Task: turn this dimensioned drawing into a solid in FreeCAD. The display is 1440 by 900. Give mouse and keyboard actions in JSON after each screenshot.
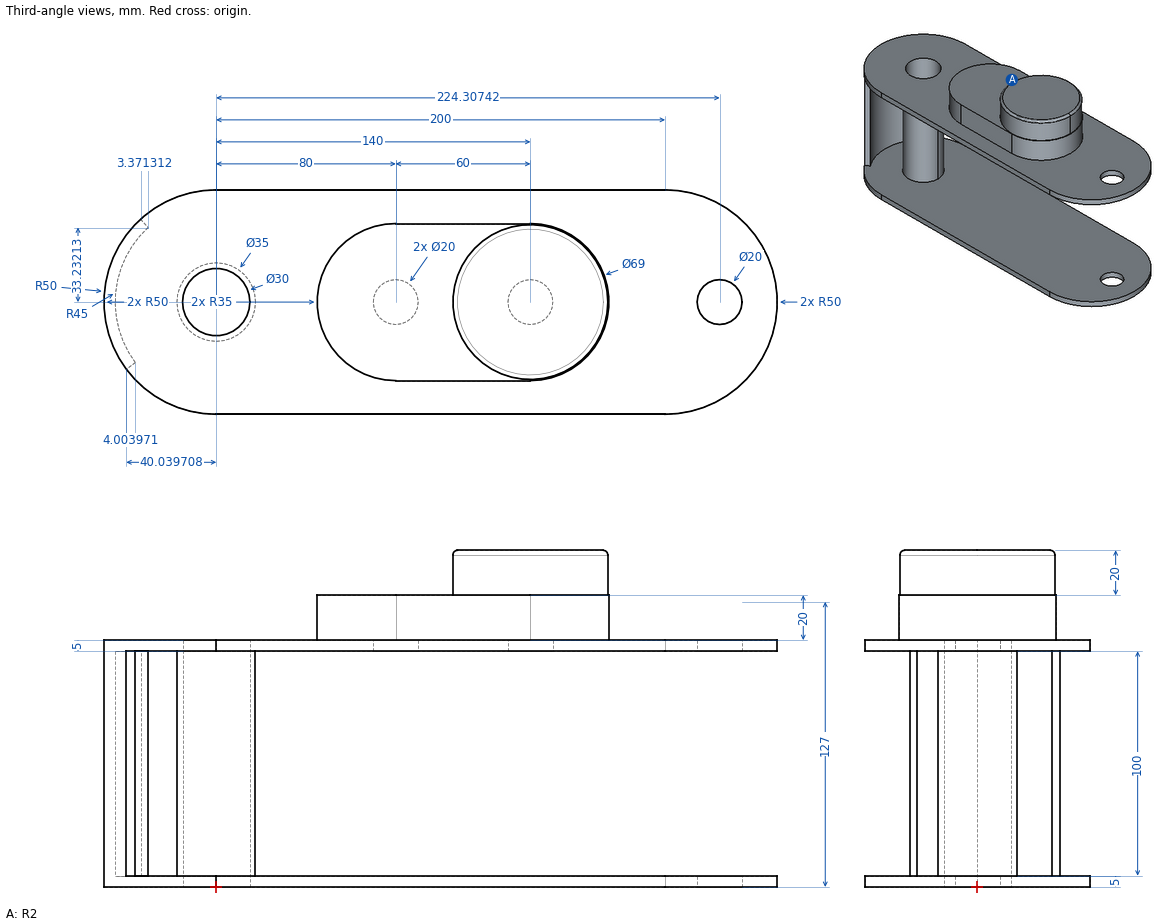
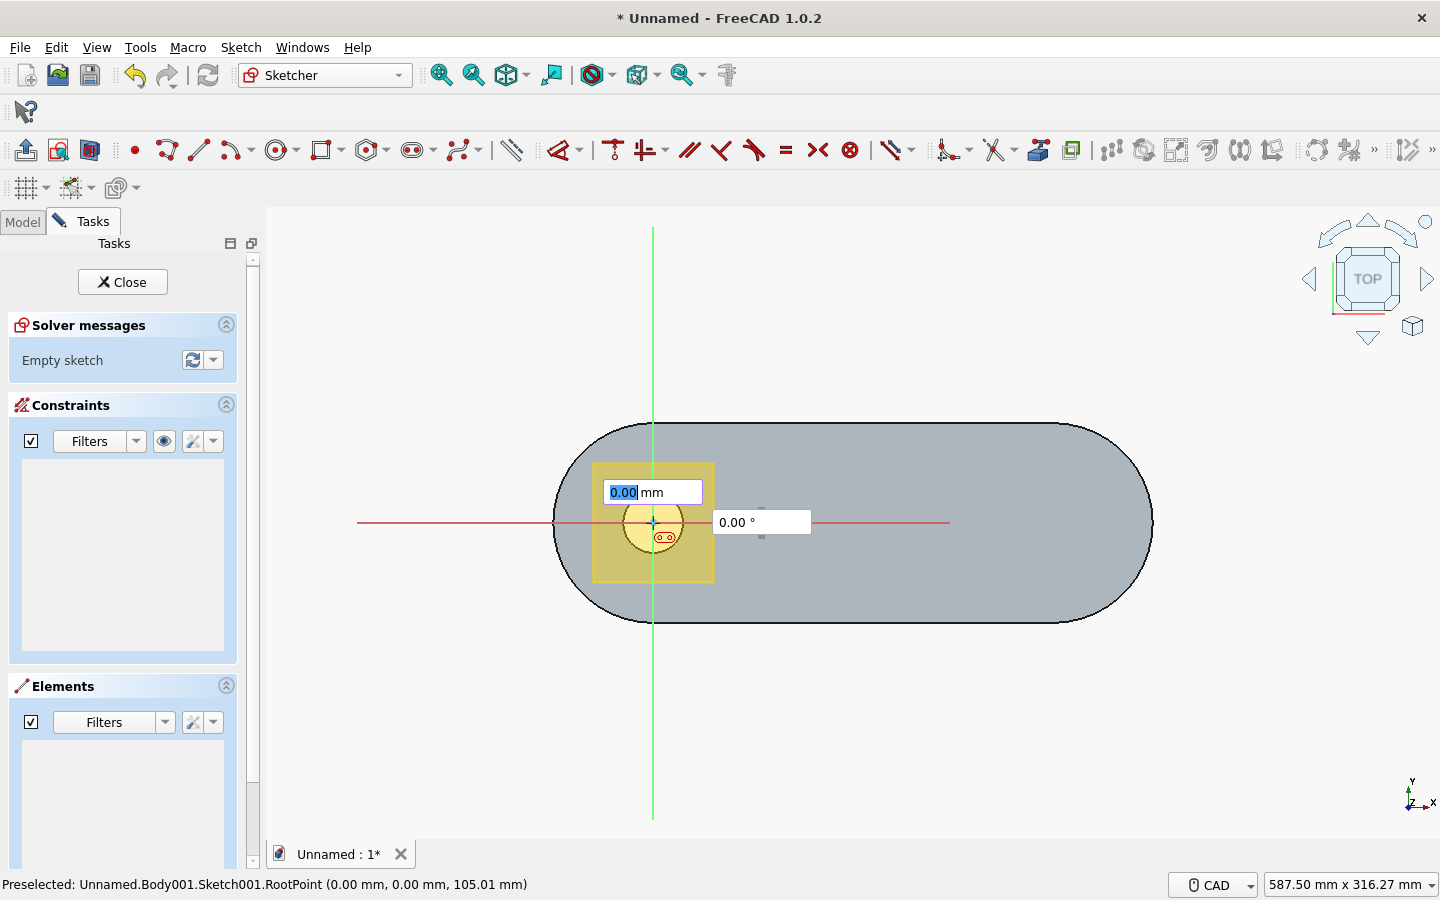
{"action": "left_click", "coordinate": [1053, 514]}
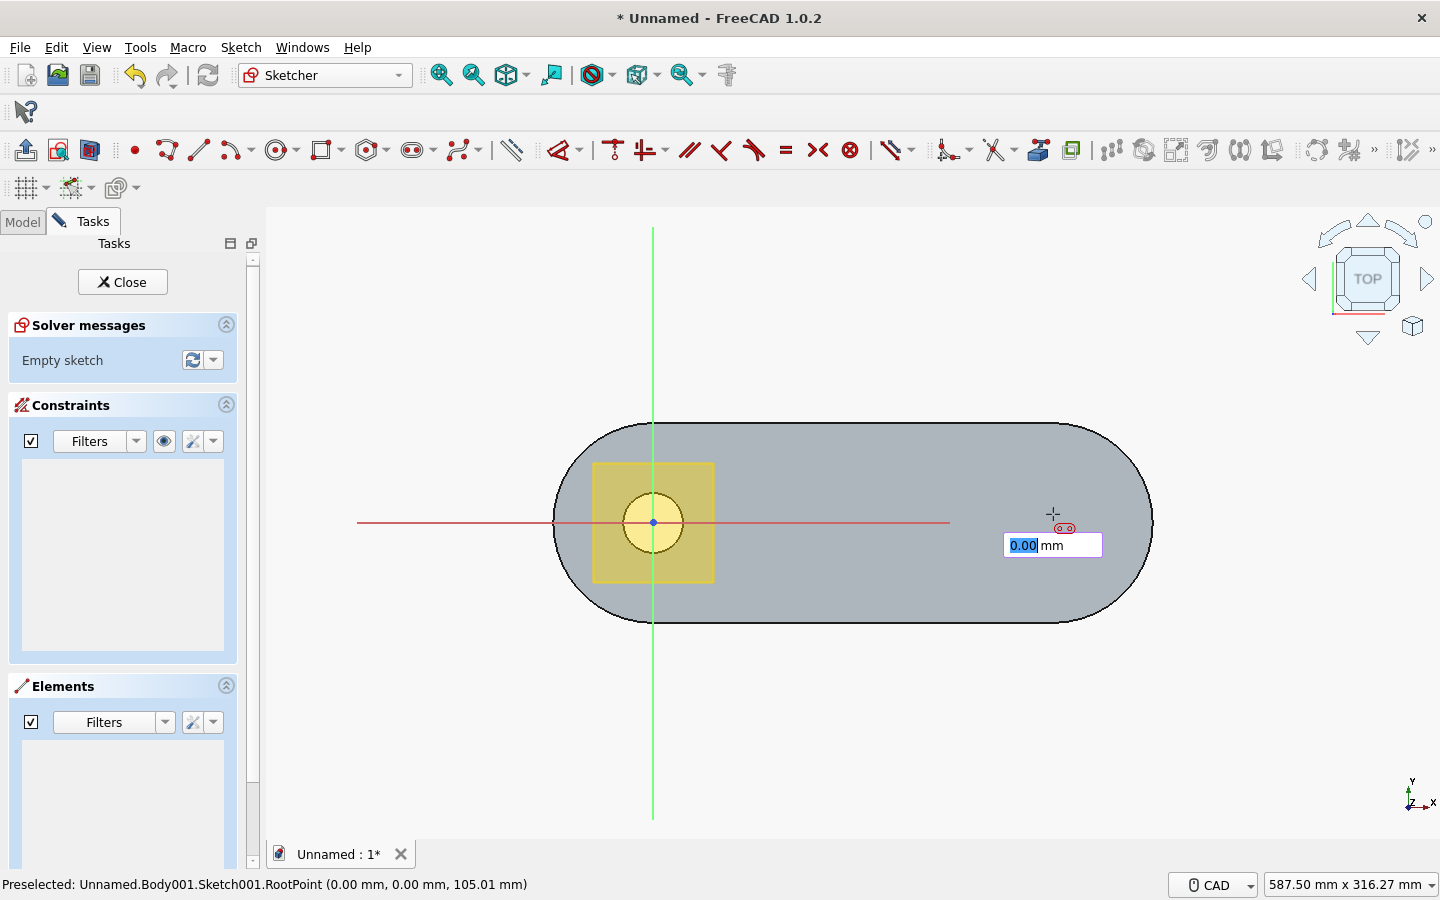
{"action": "left_click", "coordinate": [853, 623]}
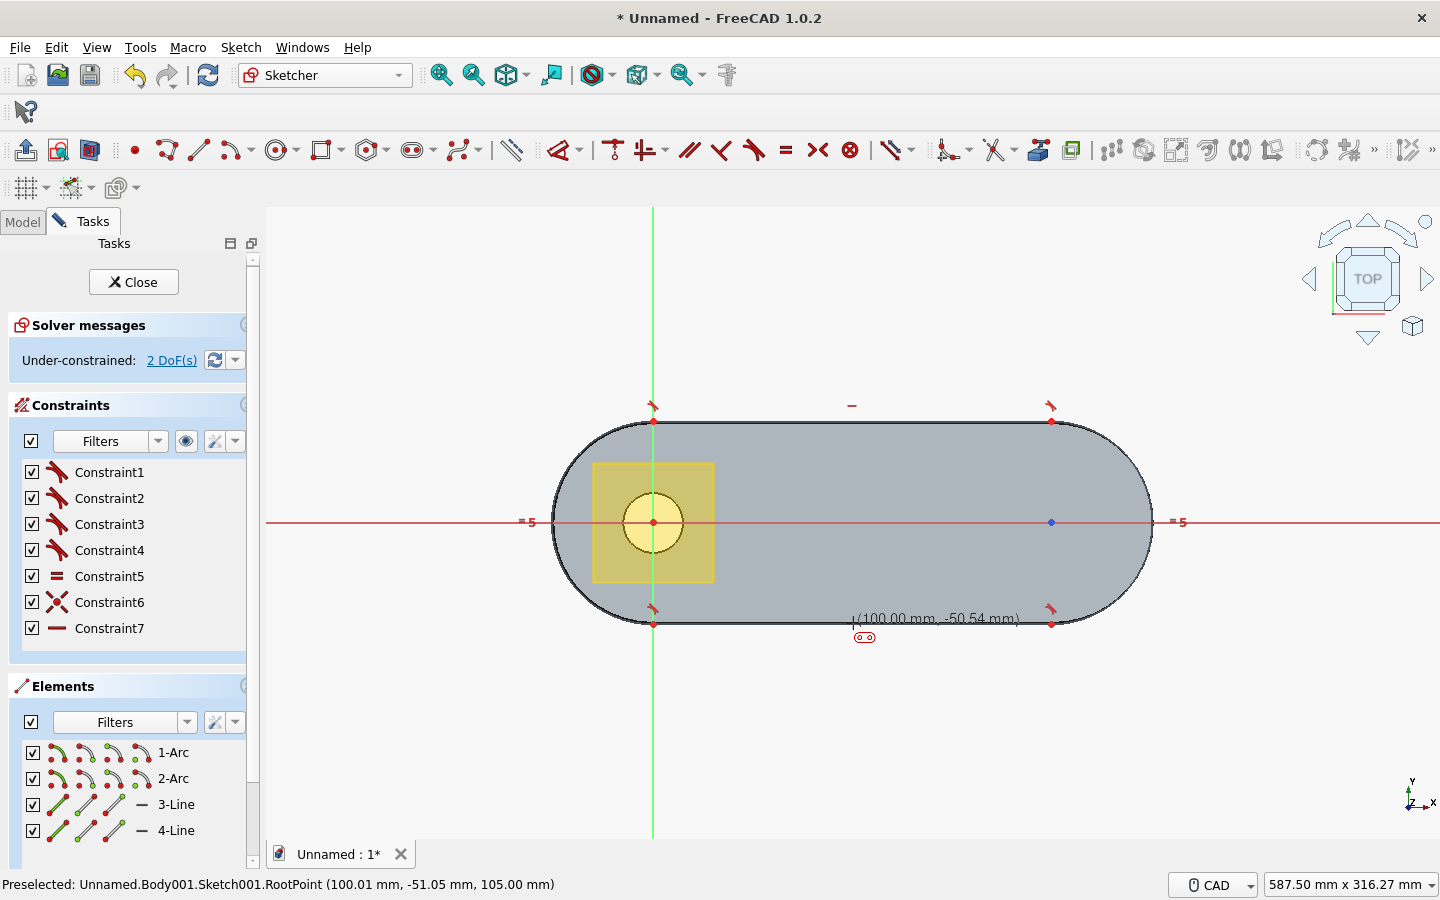
{"action": "left_click", "coordinate": [276, 150]}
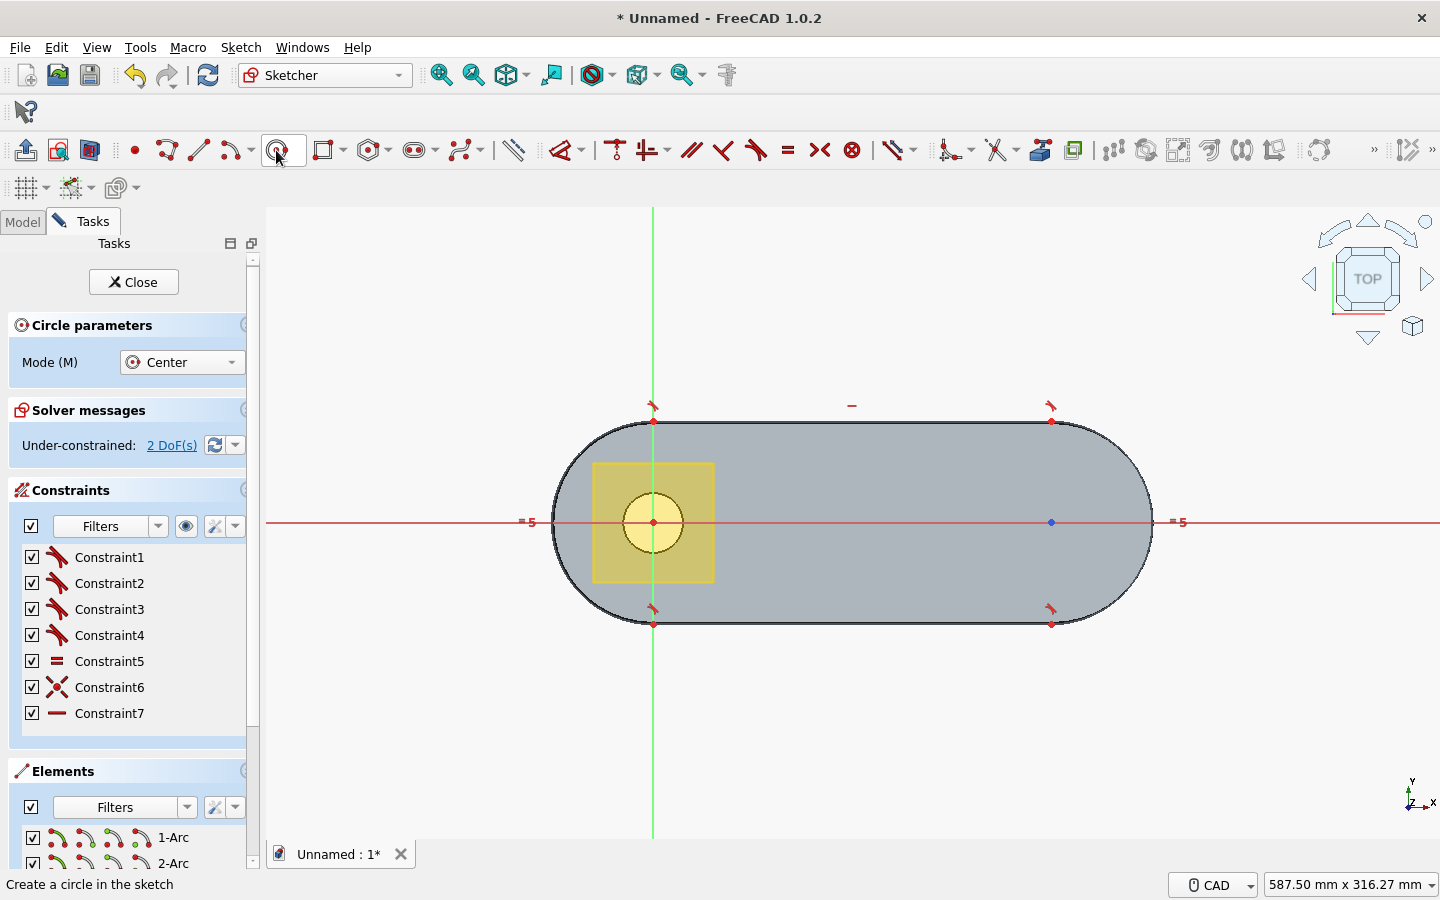
{"action": "left_click", "coordinate": [653, 523]}
{"action": "left_click", "coordinate": [674, 502]}
{"action": "key", "text": "Escape"}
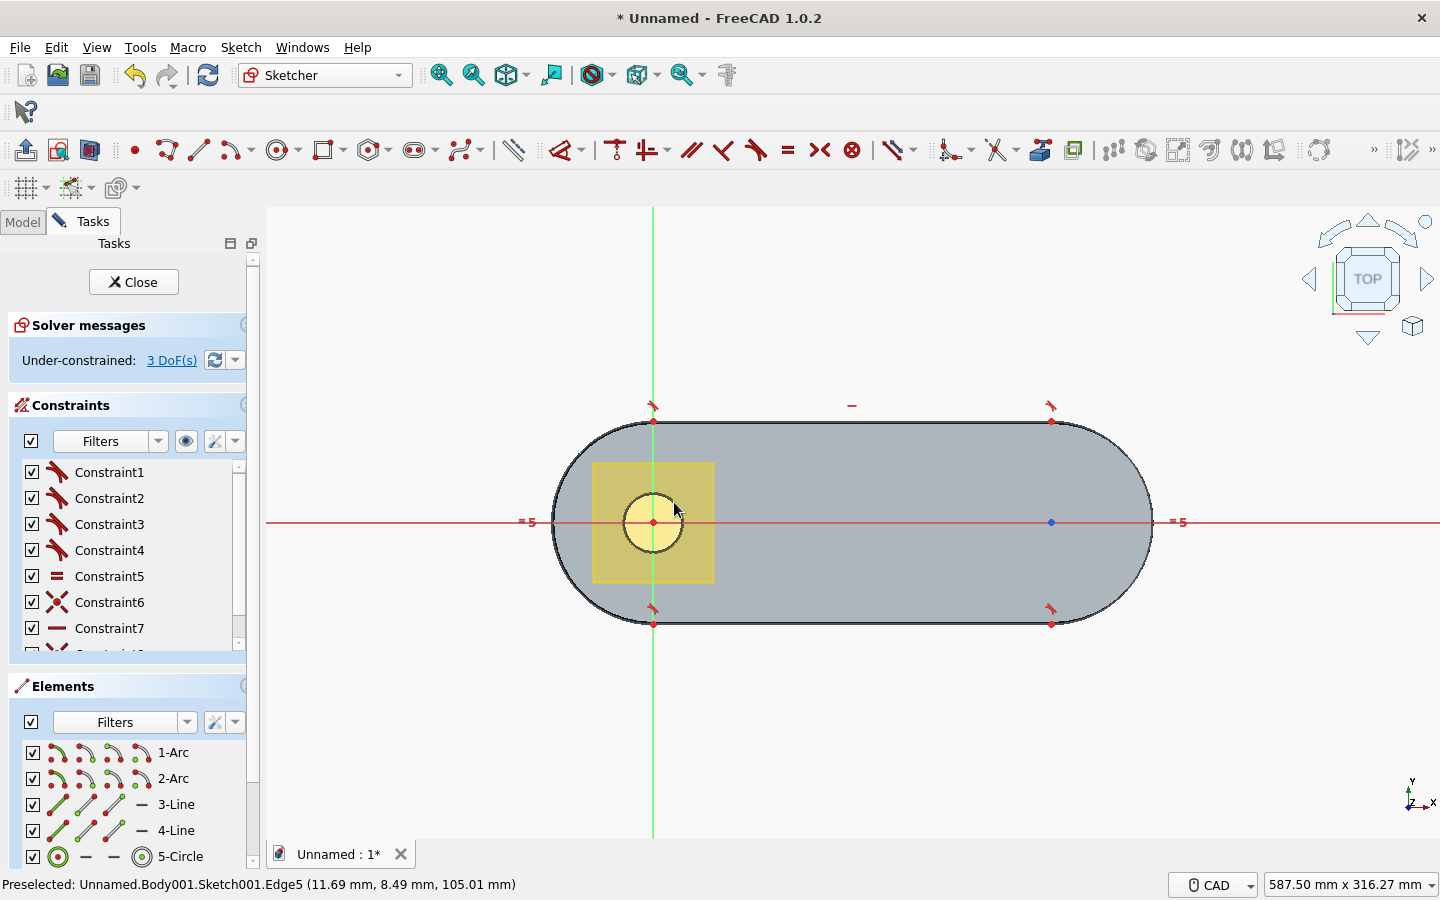
{"action": "left_click", "coordinate": [560, 150]}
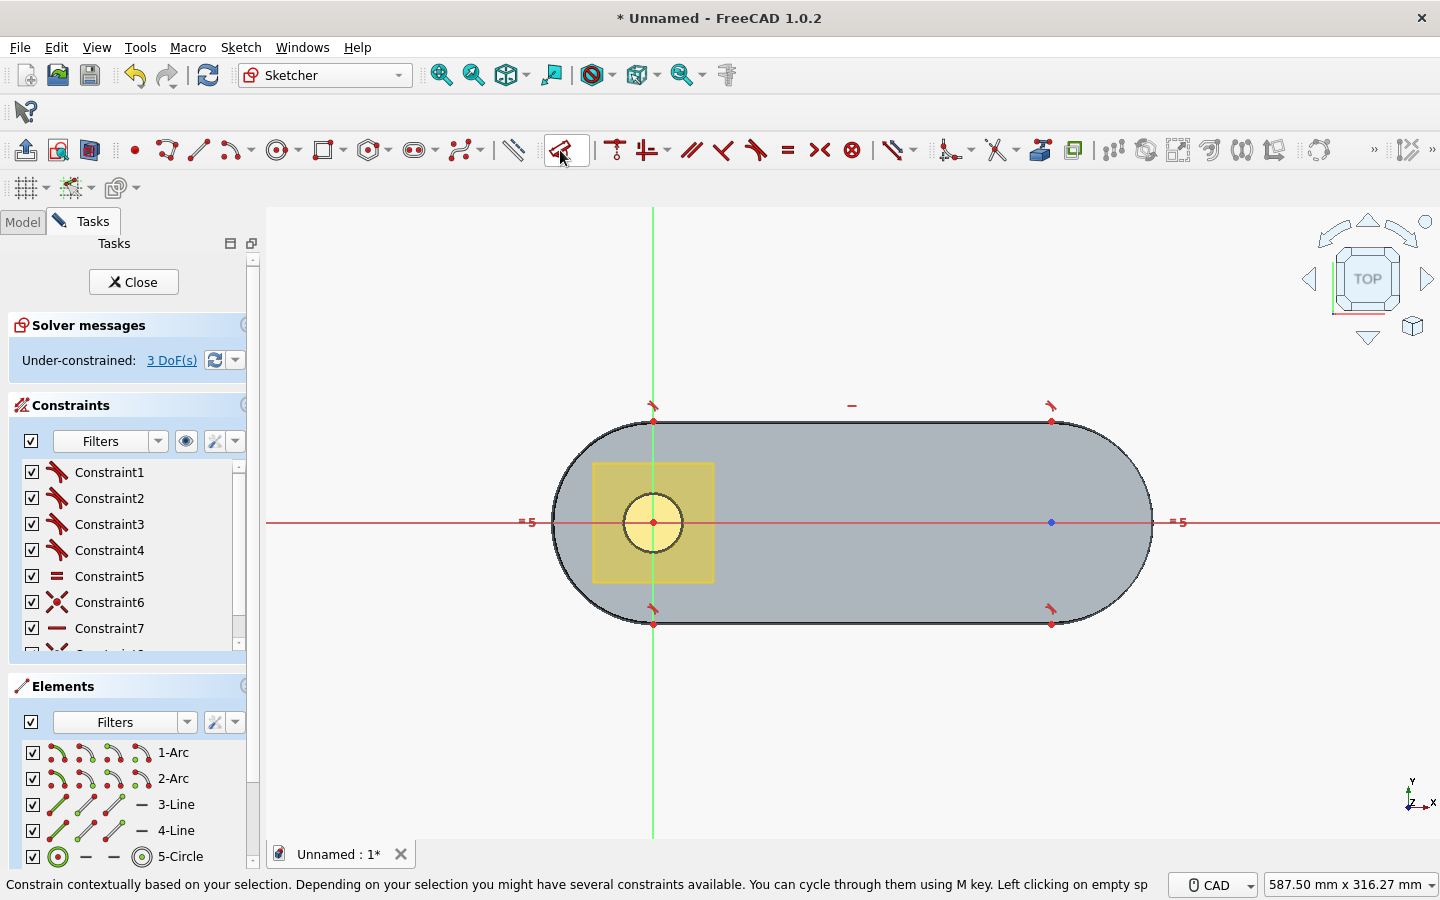
{"action": "left_click", "coordinate": [571, 463]}
{"action": "left_click", "coordinate": [545, 444]}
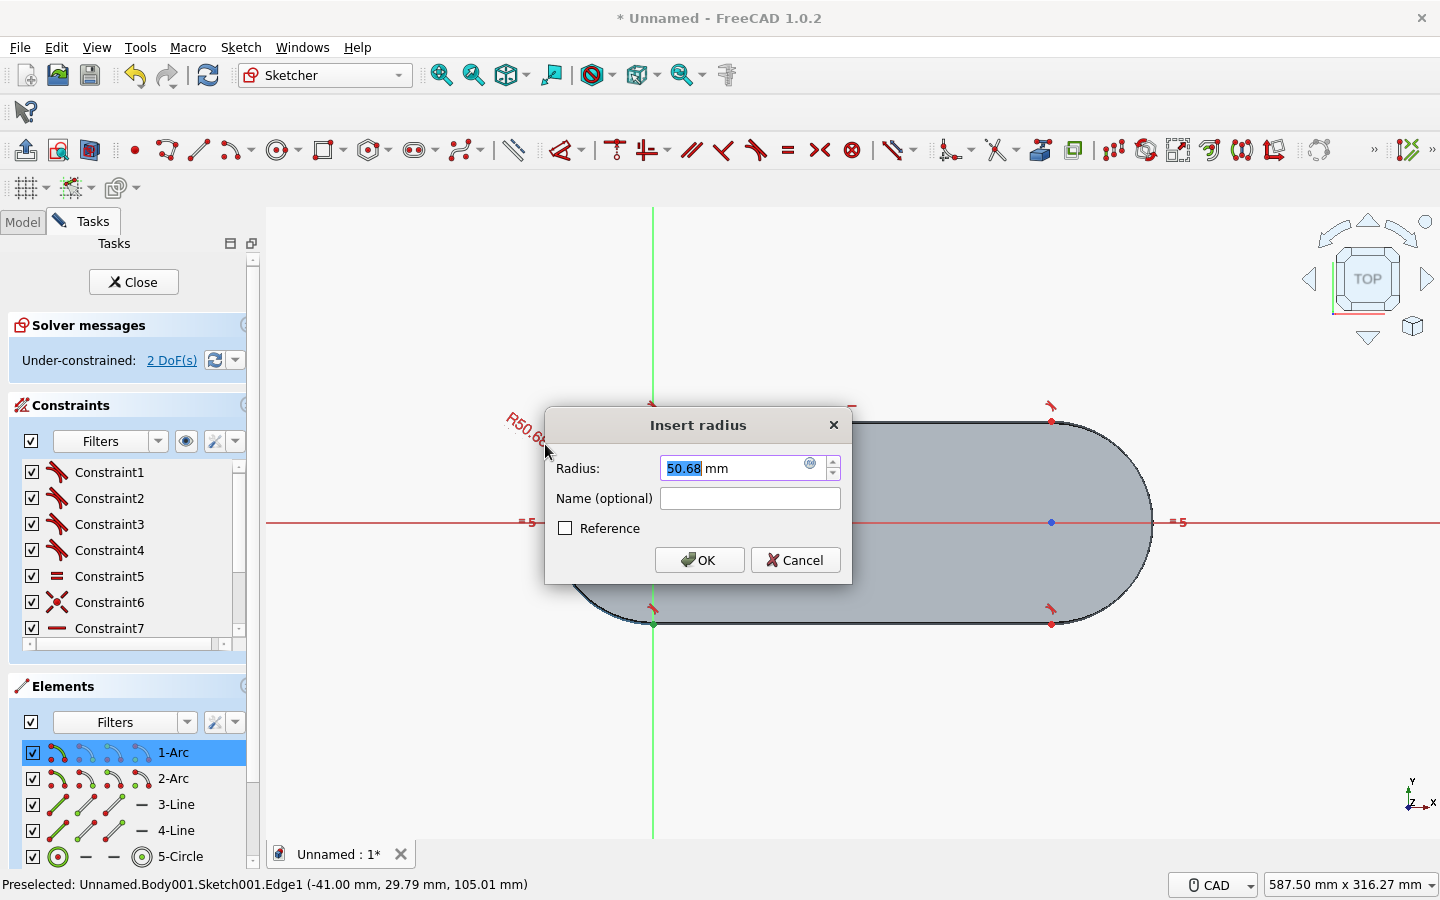
{"action": "type", "text": "50"}
{"action": "key", "text": "Return"}